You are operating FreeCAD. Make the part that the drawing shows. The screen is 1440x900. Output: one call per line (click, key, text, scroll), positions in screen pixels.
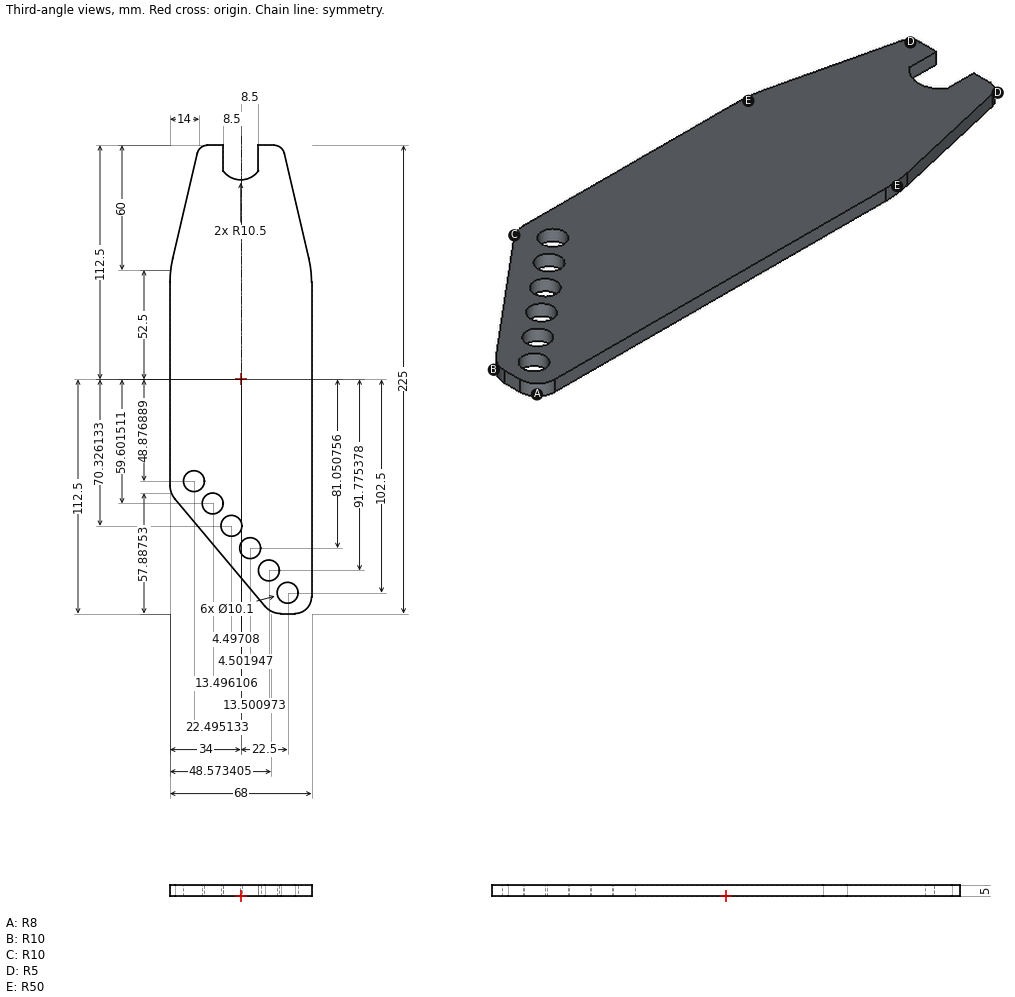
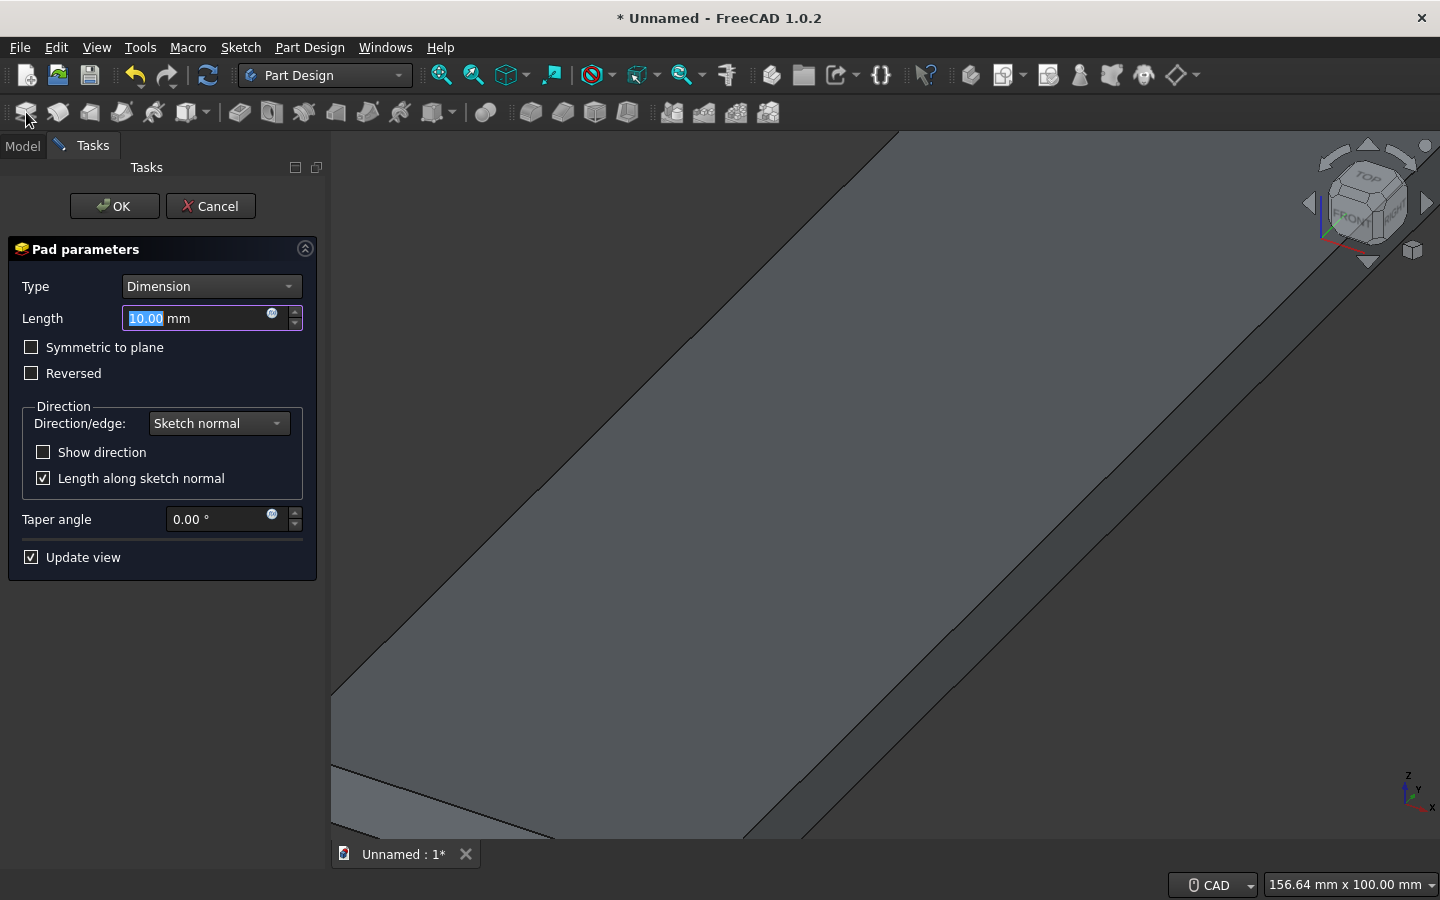
text(5)
key(Tab)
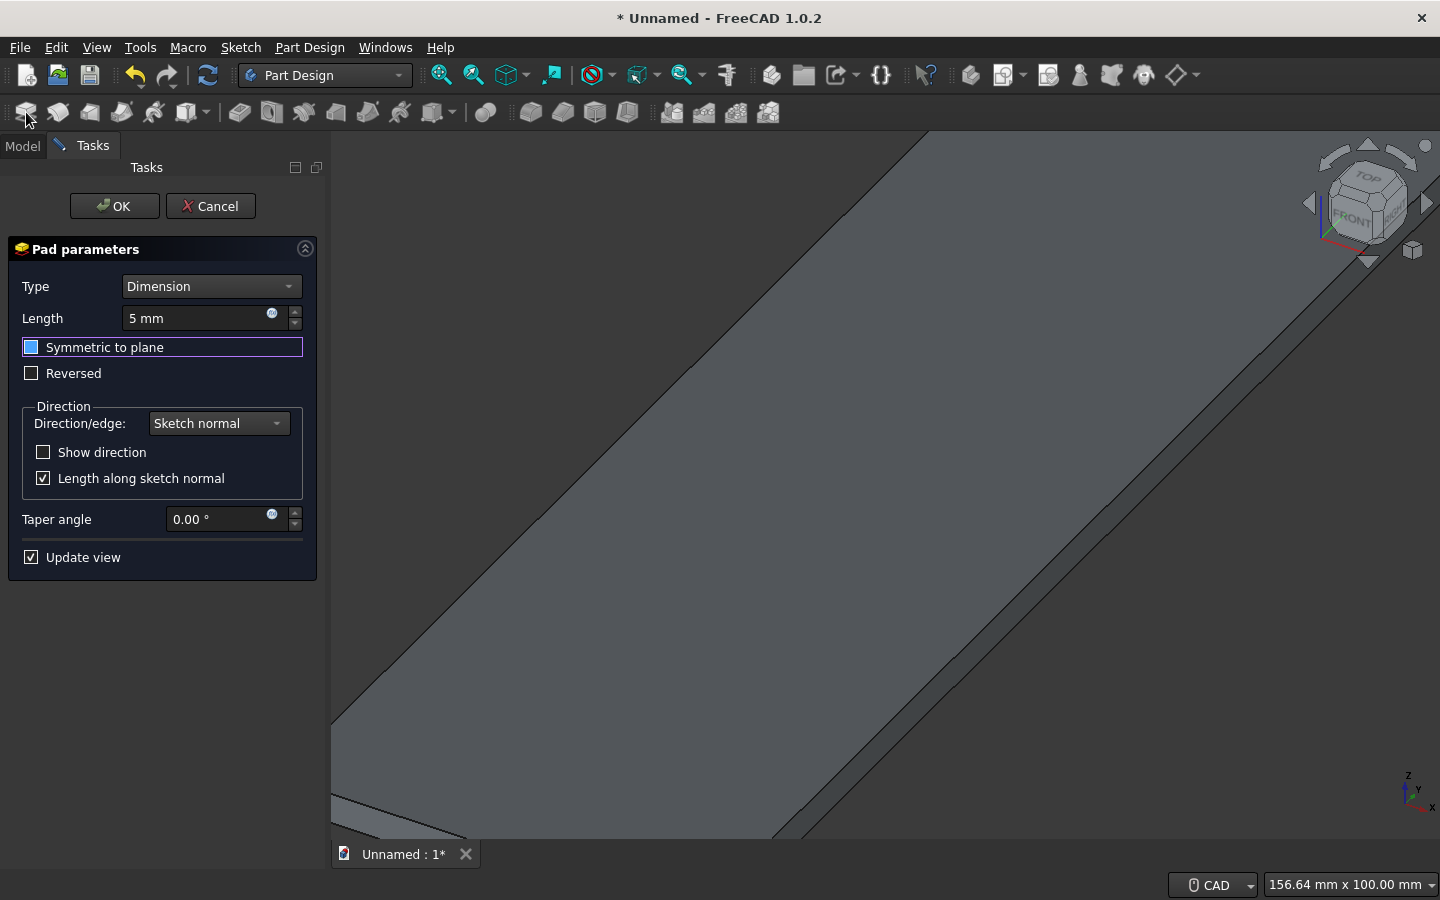
click(115, 206)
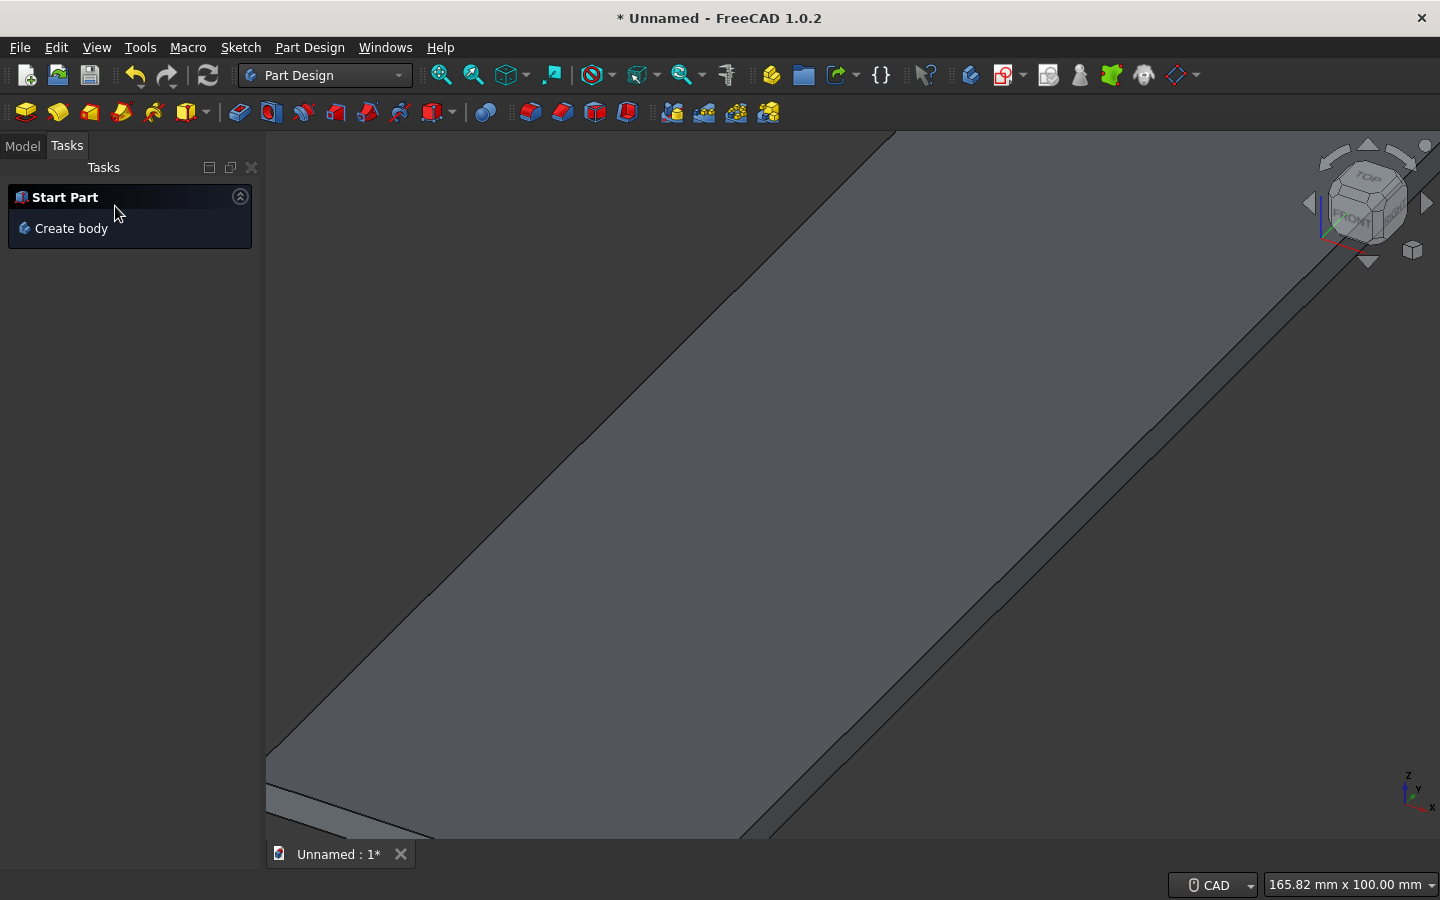
click(442, 76)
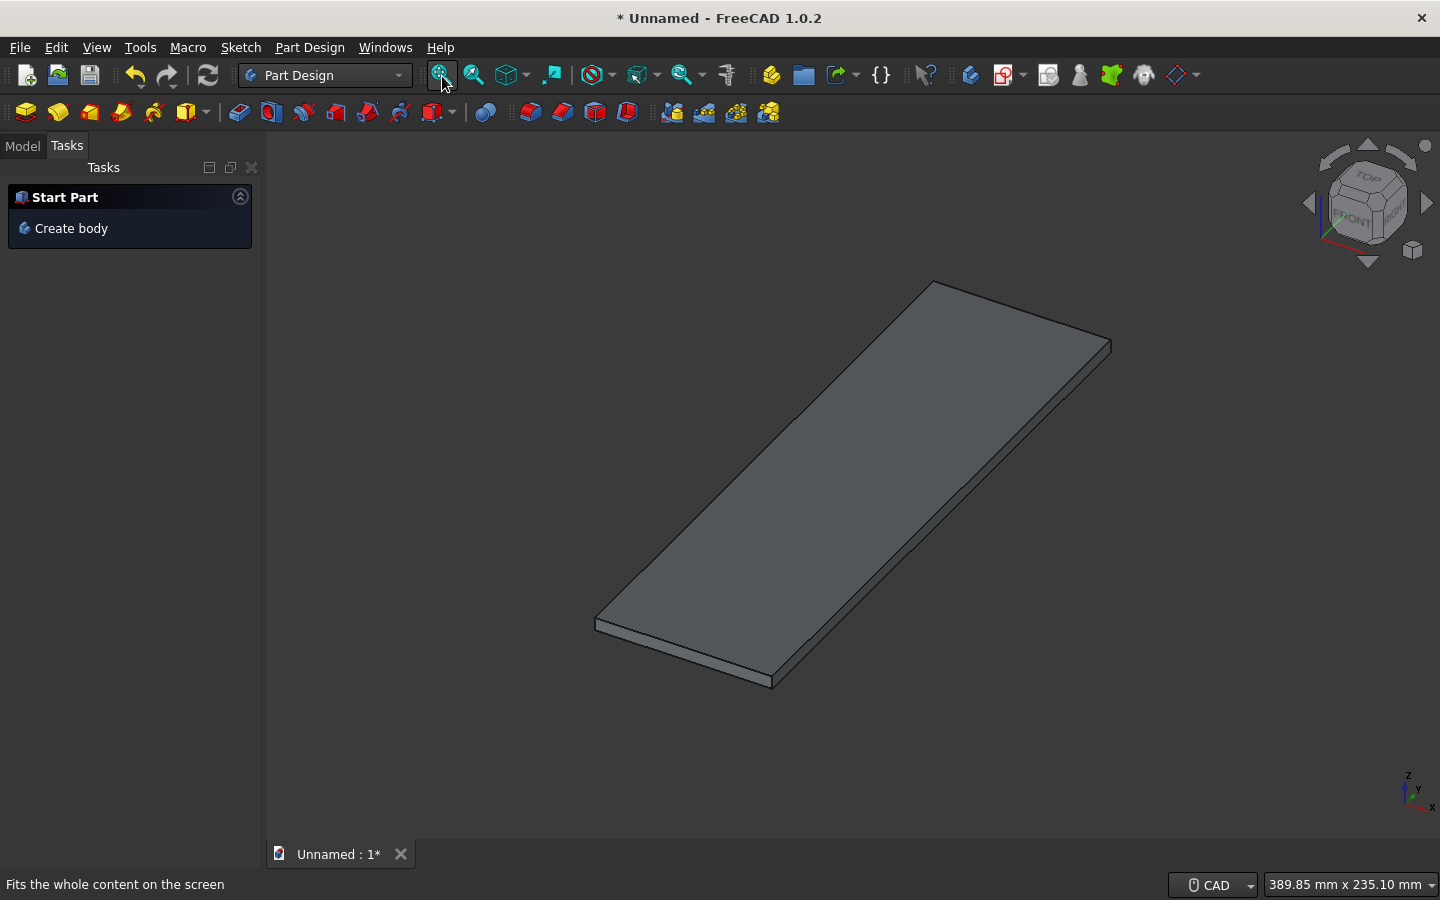
click(950, 382)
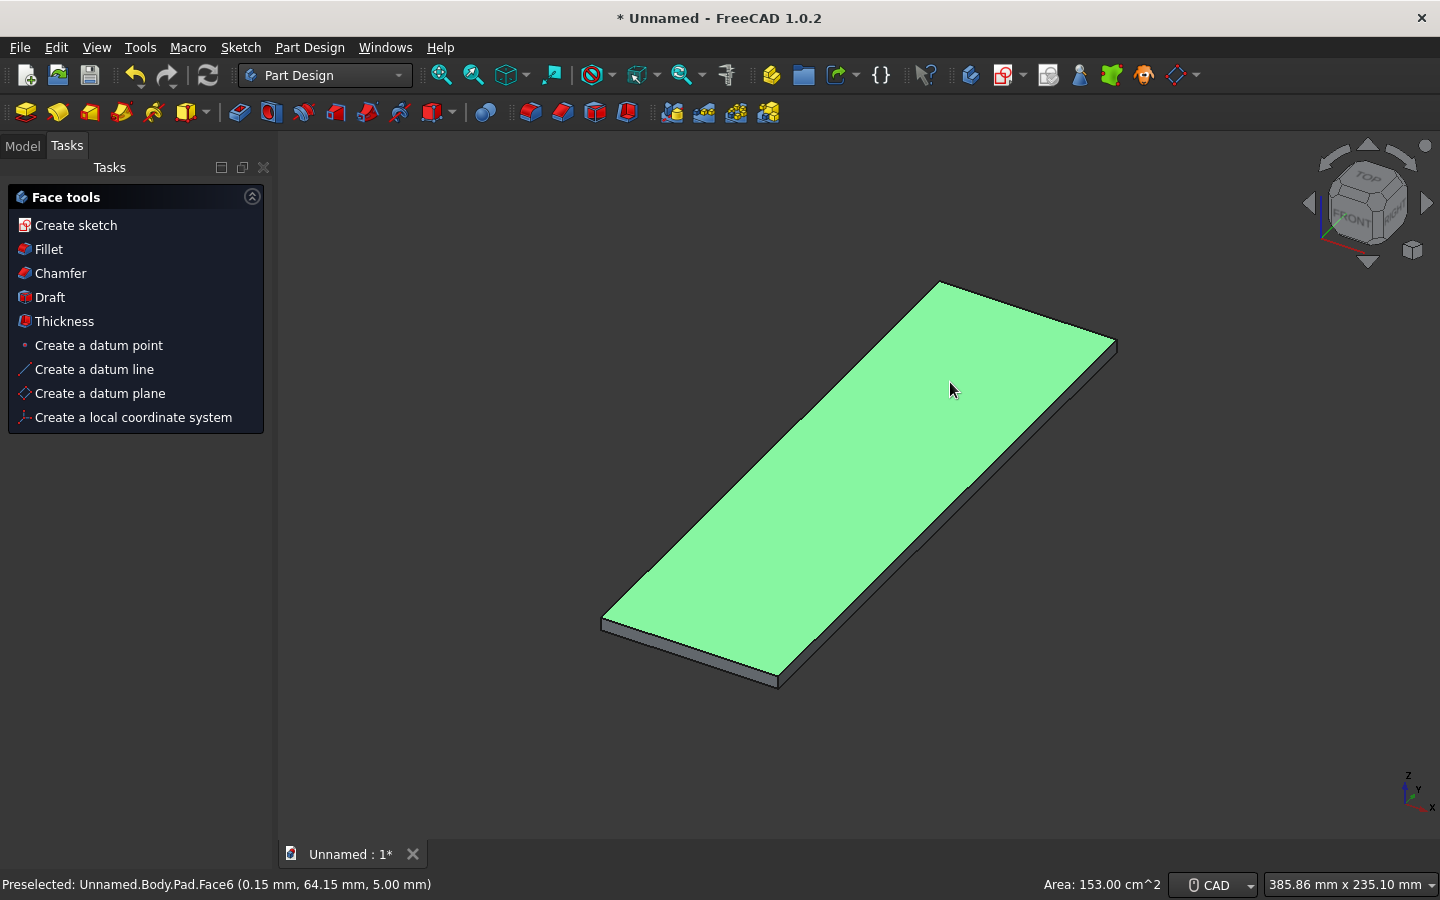
click(1004, 76)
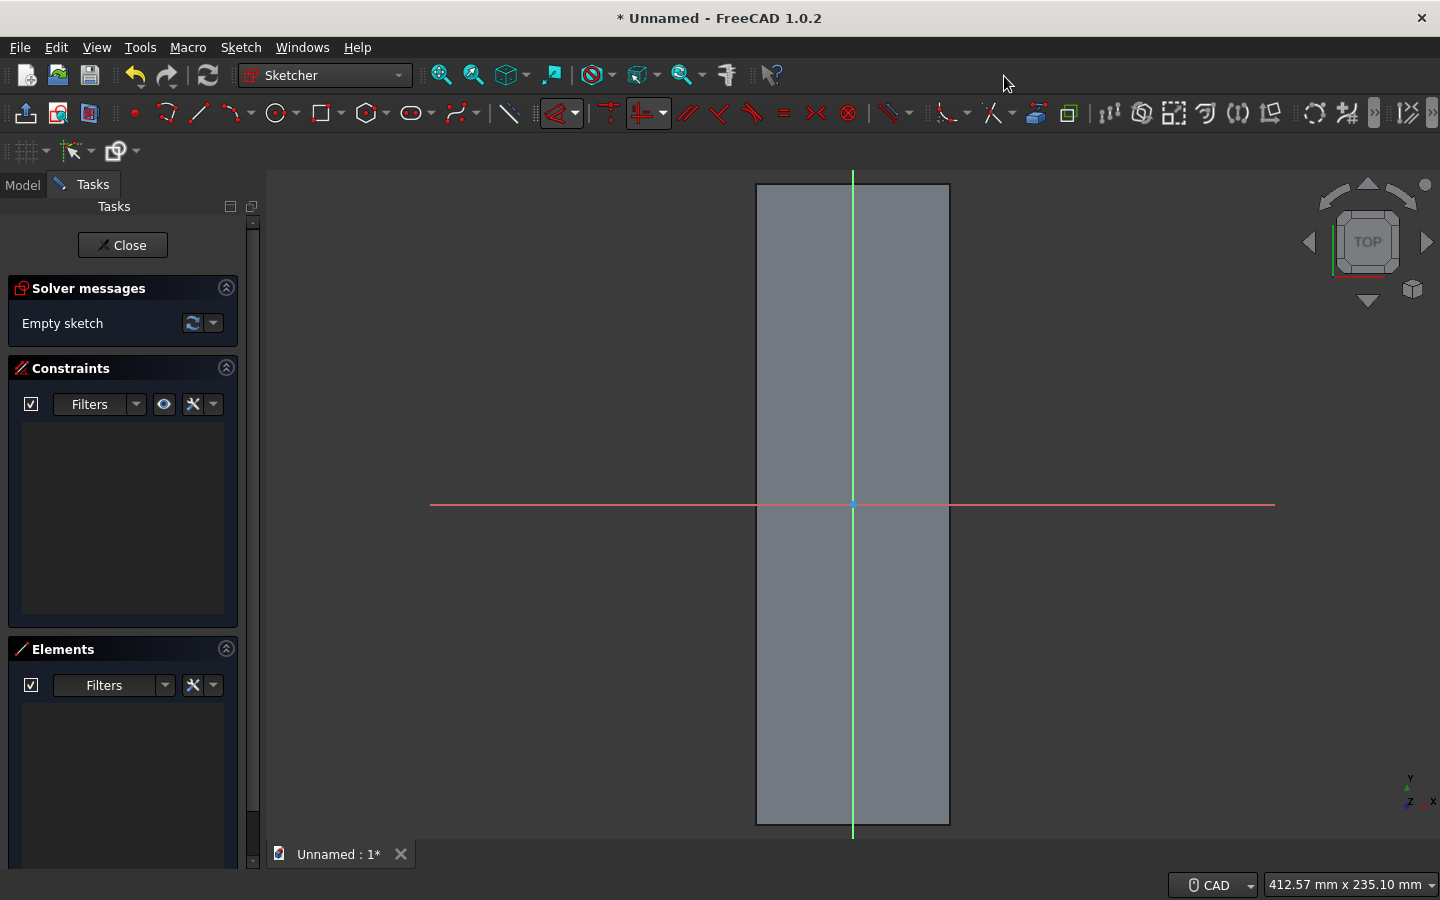
scroll(475, 198, down, 1)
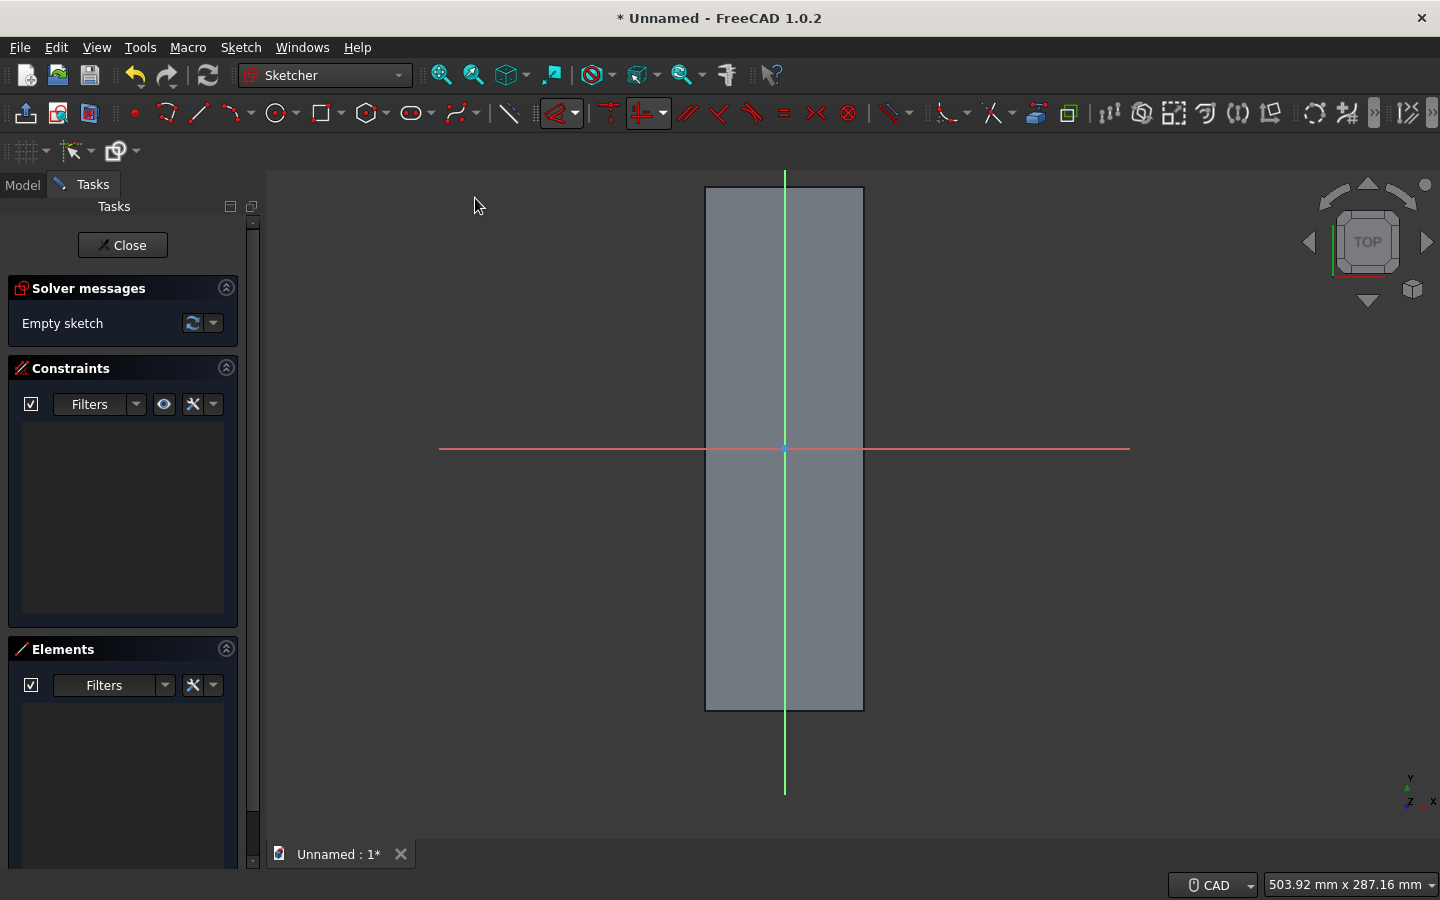
scroll(785, 659, up, 3)